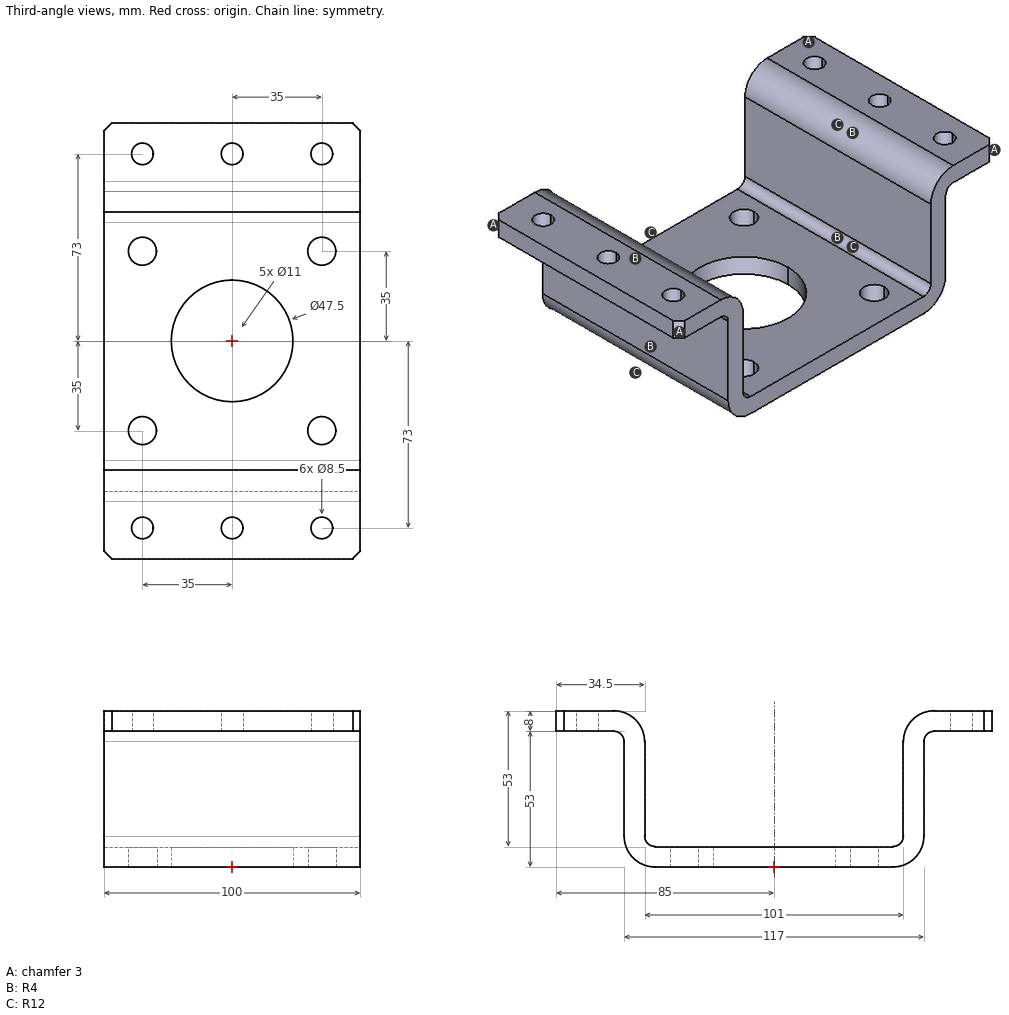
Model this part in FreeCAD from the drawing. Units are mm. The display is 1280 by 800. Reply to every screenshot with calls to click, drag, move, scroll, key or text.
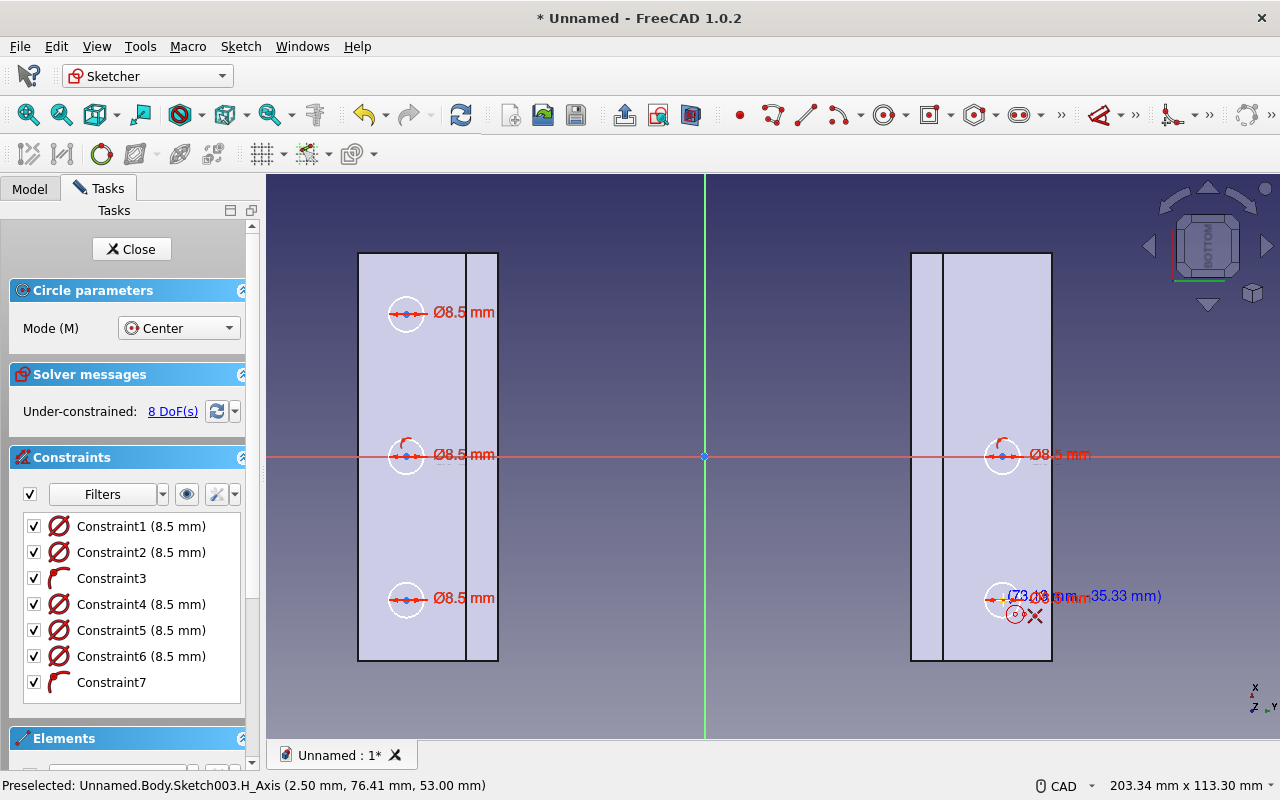
scroll(1003, 314, up, 2)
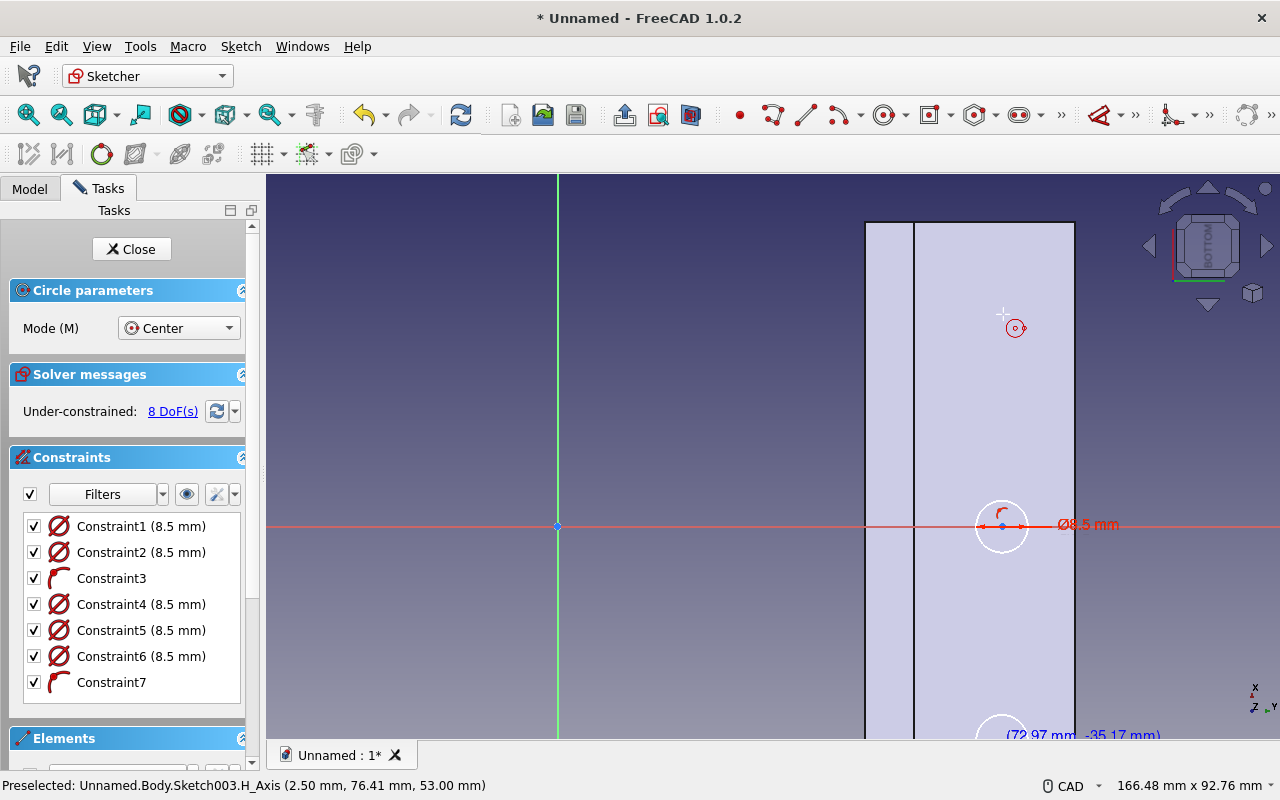
click(1002, 314)
move(1020, 295)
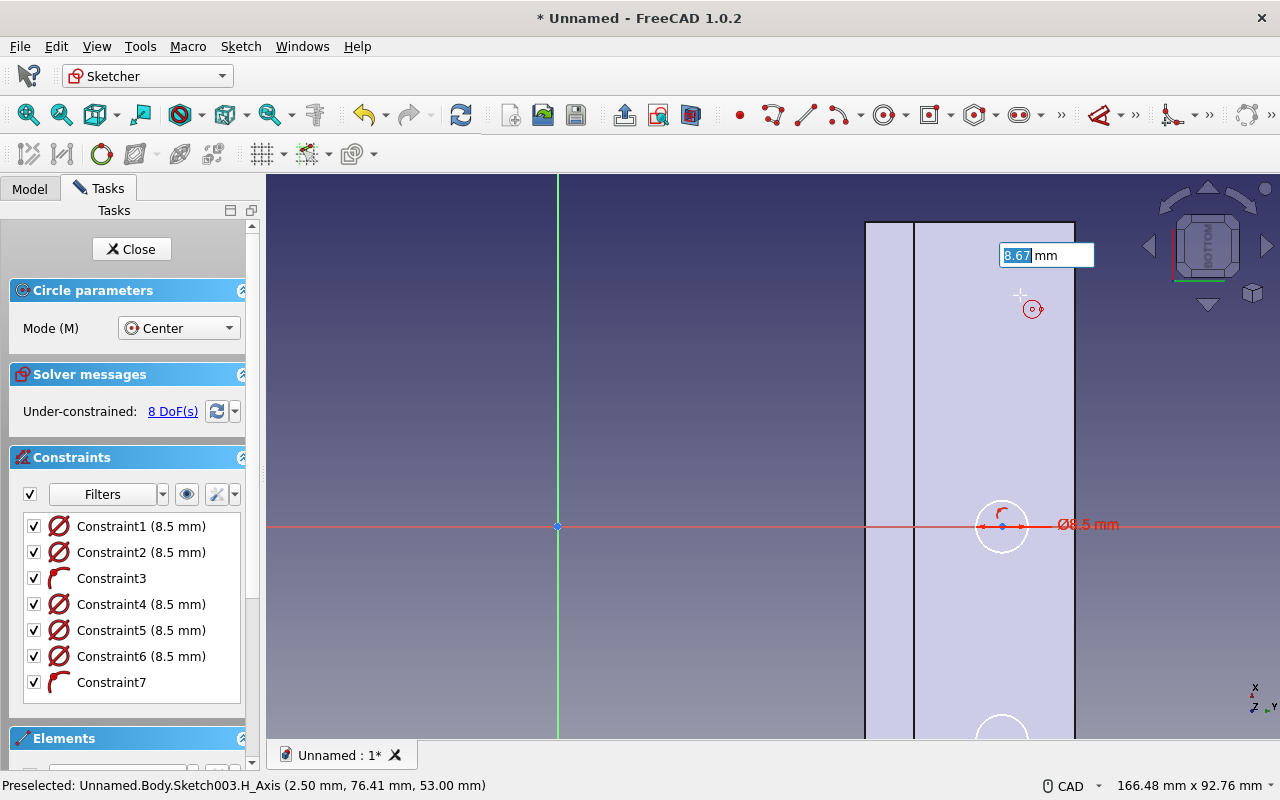
text(8.5)
key(Return)
key(Escape)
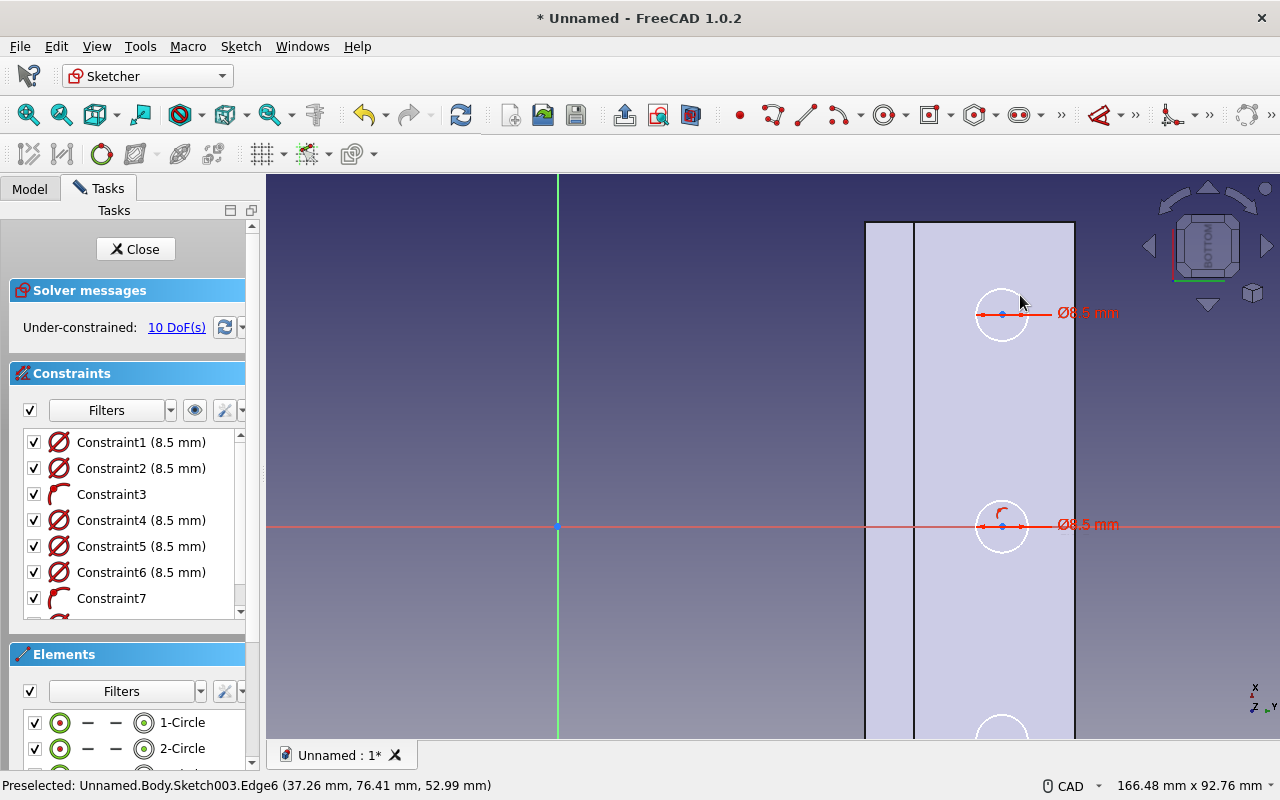
scroll(1003, 314, down, 2)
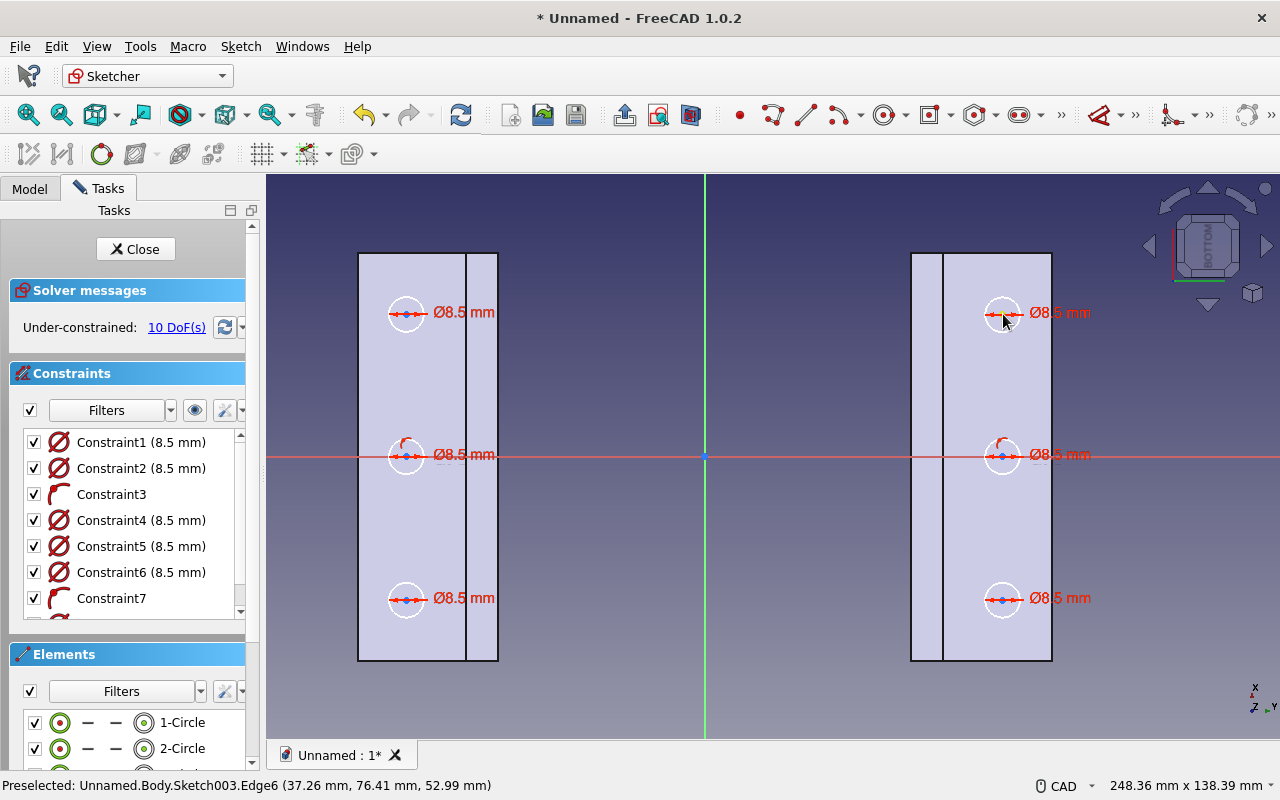
click(406, 314)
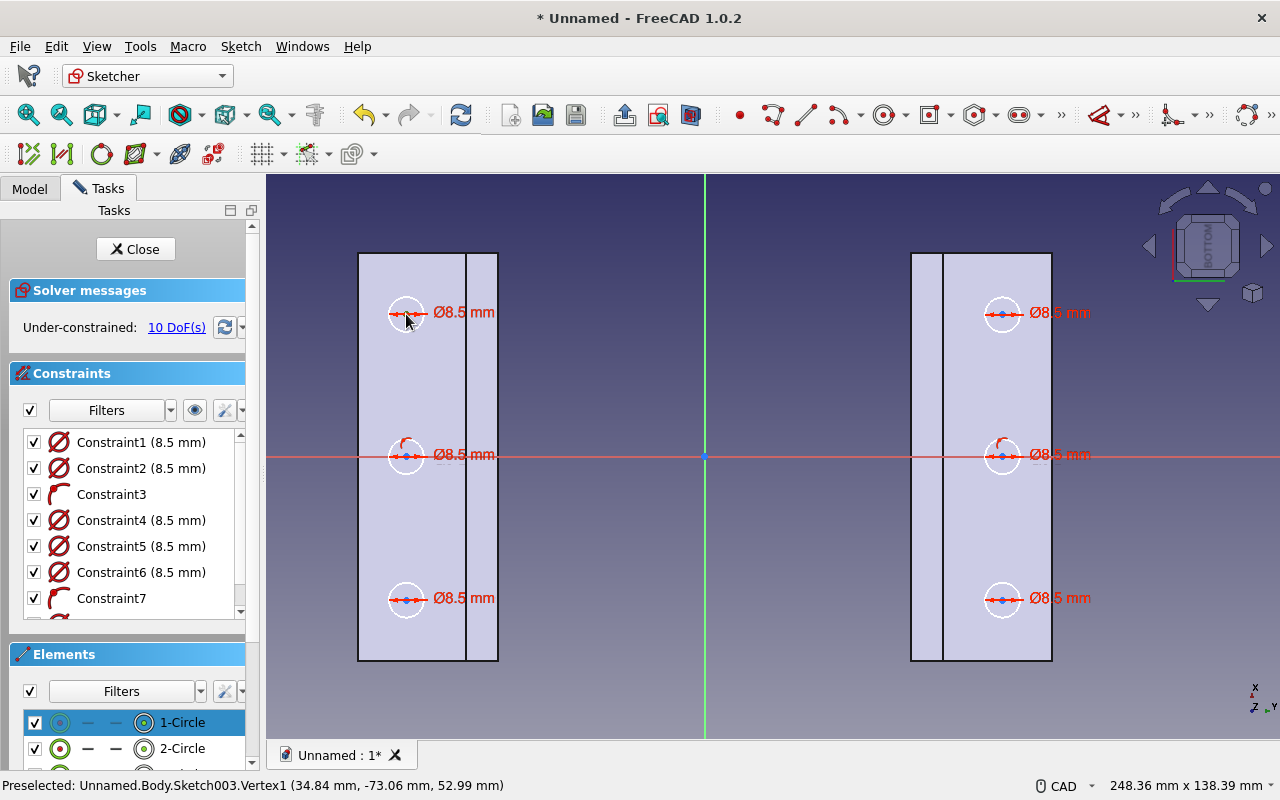
click(406, 457)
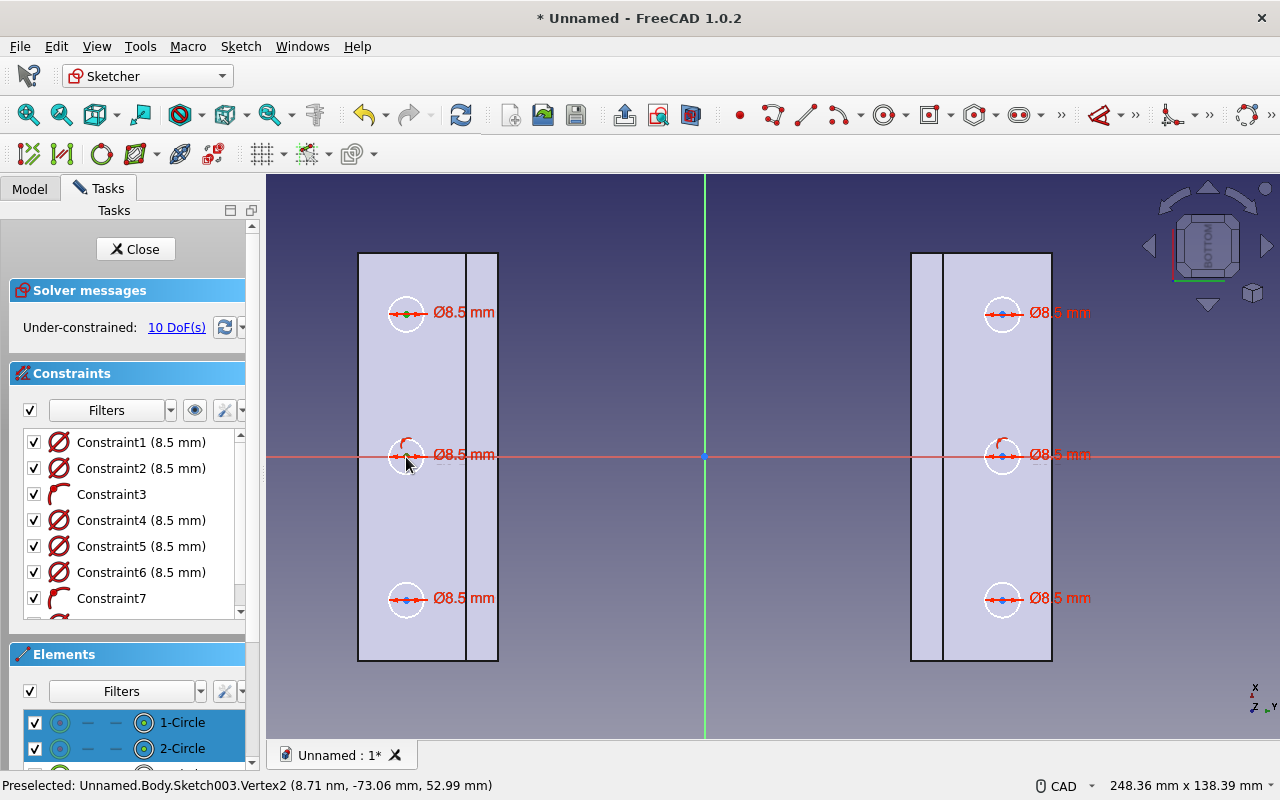
key(v)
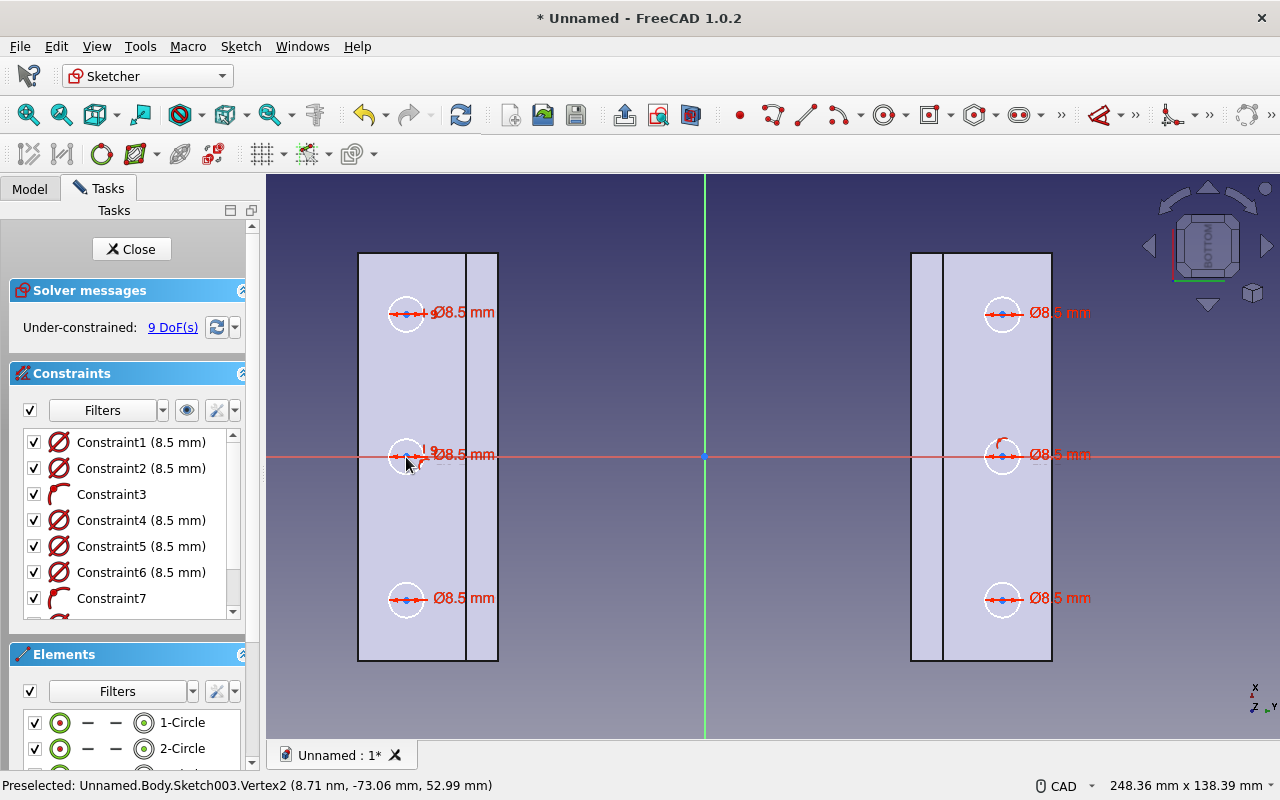
click(406, 457)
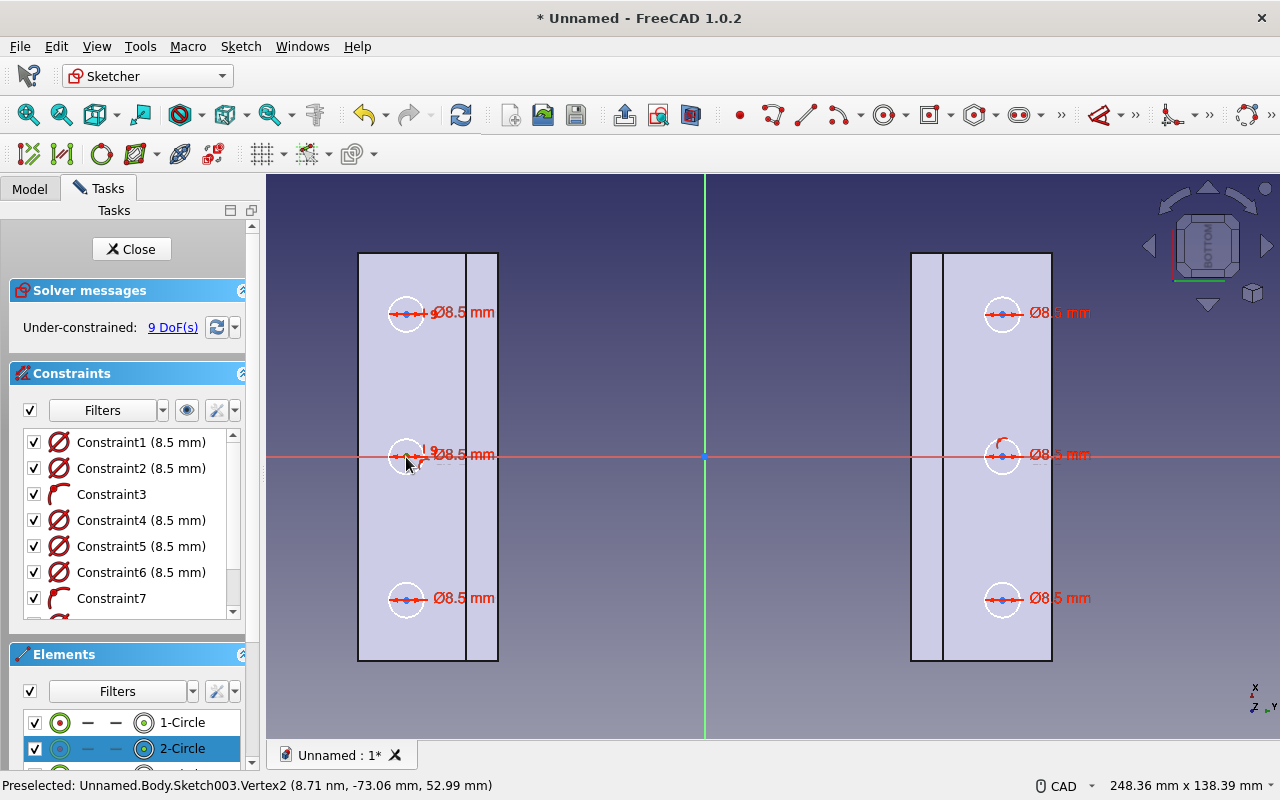
click(406, 600)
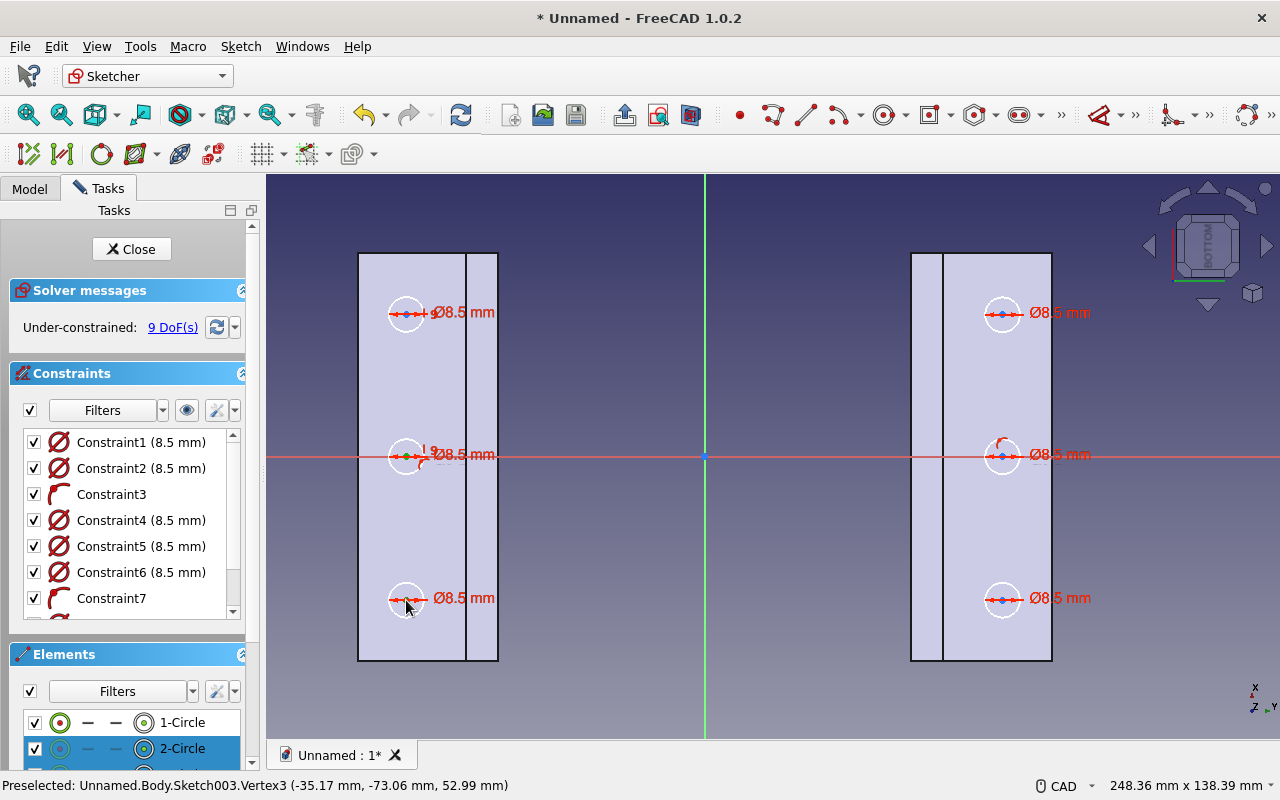
key(v)